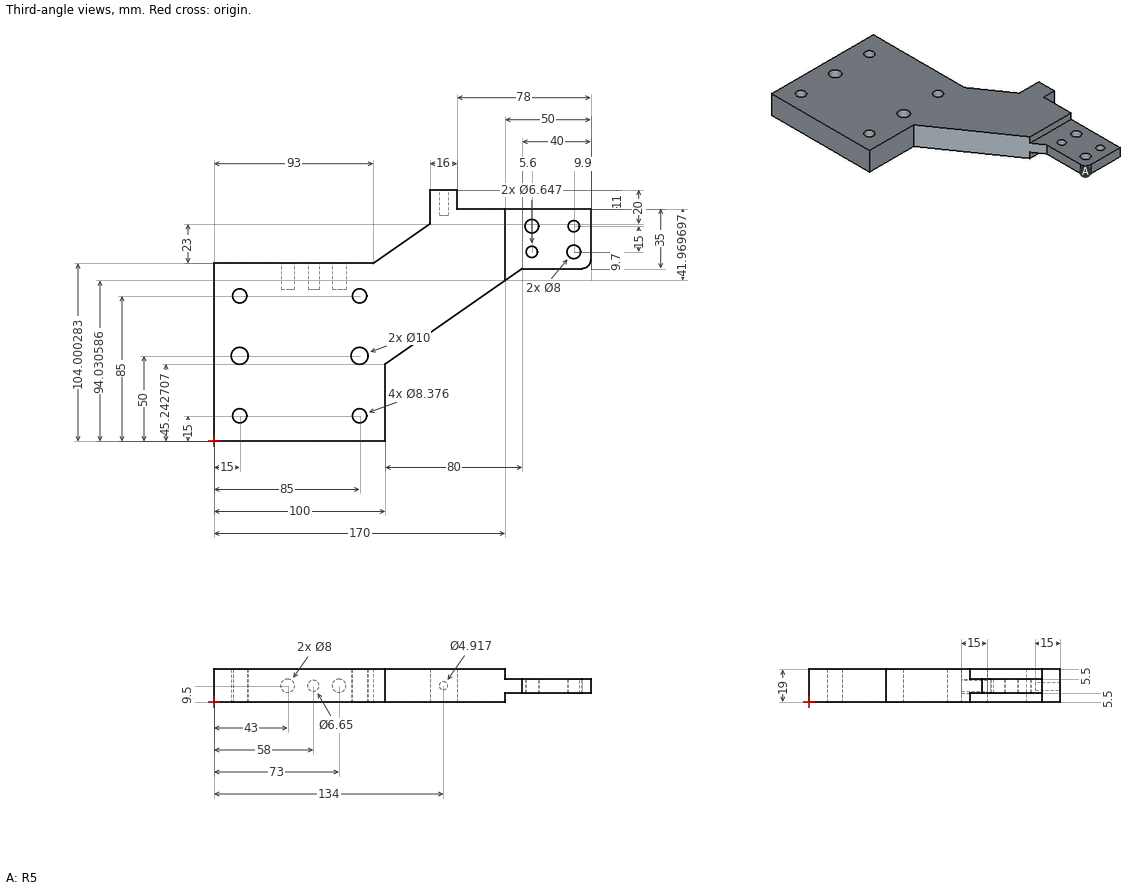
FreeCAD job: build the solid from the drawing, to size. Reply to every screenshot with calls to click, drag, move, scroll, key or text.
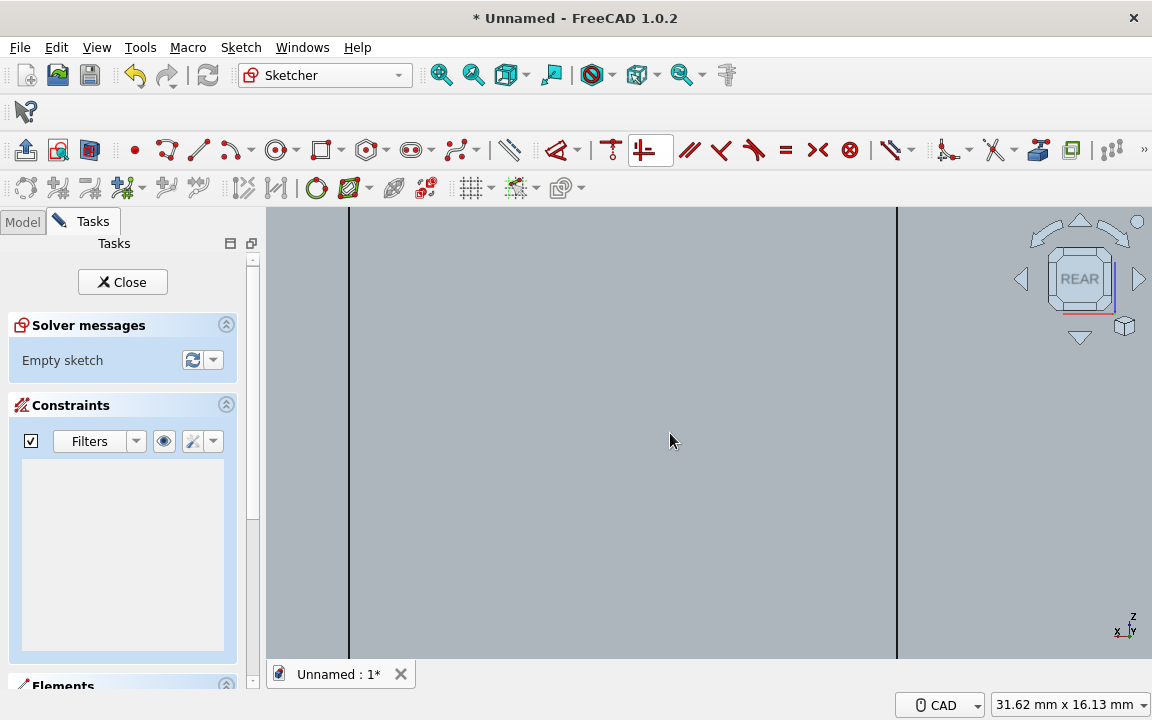
scroll(602, 412, up, 3)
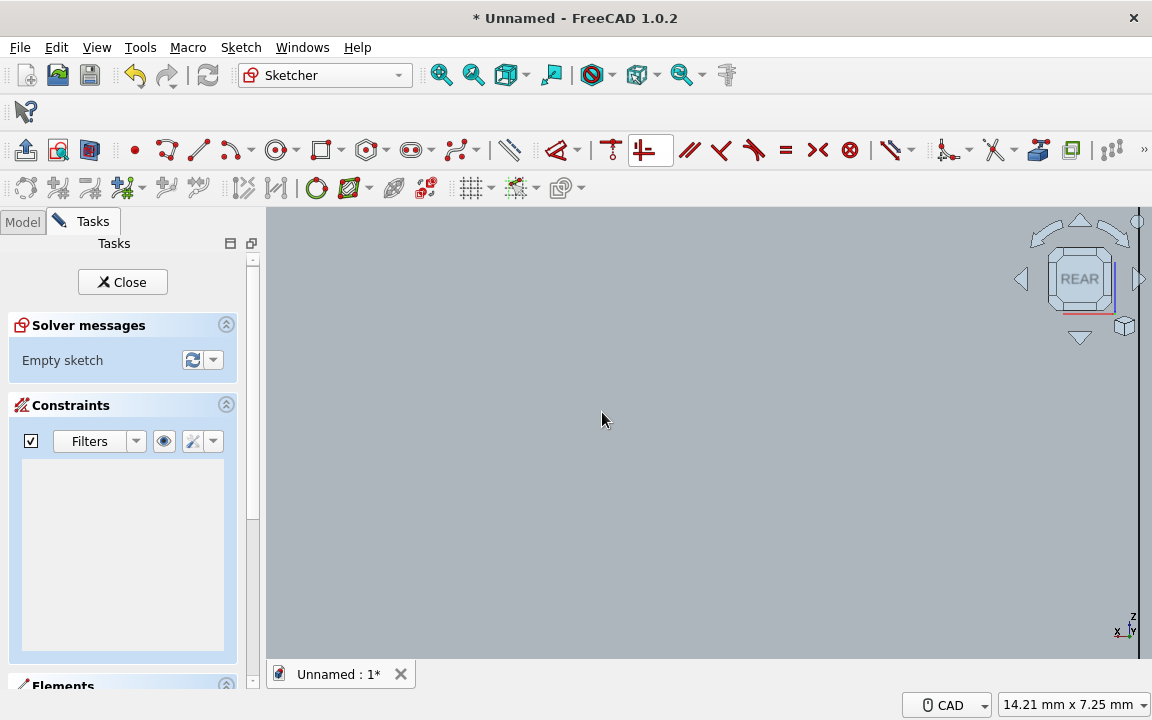
click(276, 150)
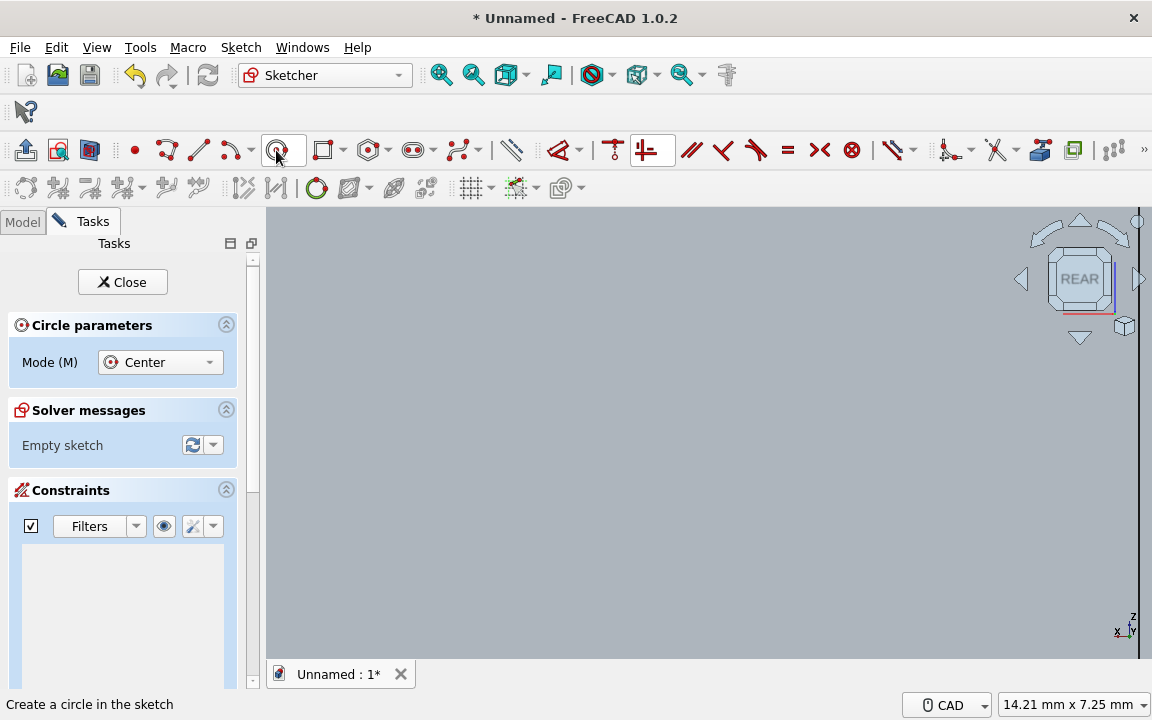
click(640, 432)
click(749, 324)
key(Escape)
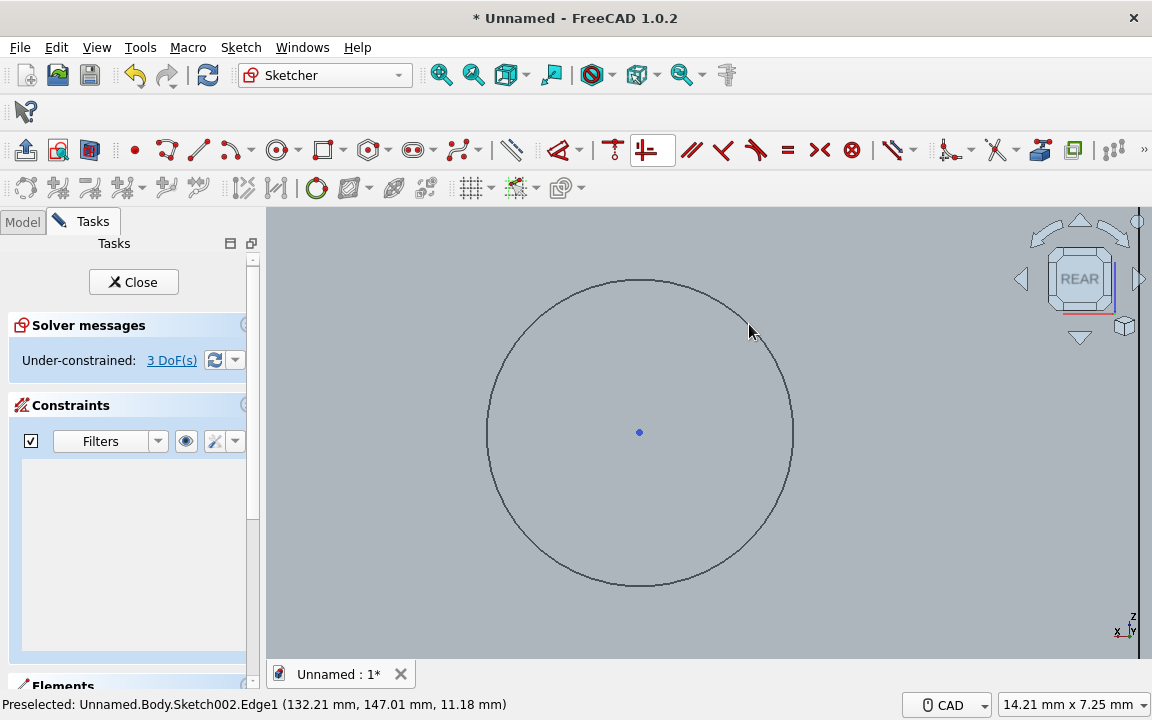
click(558, 150)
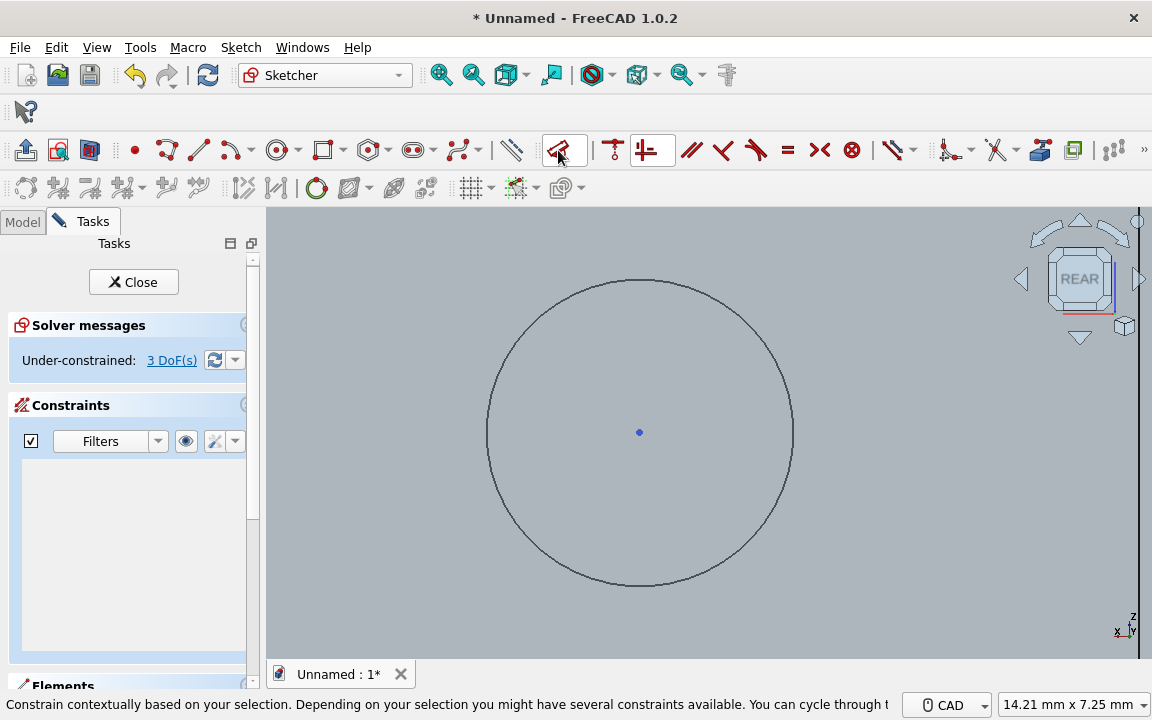
click(748, 324)
click(771, 301)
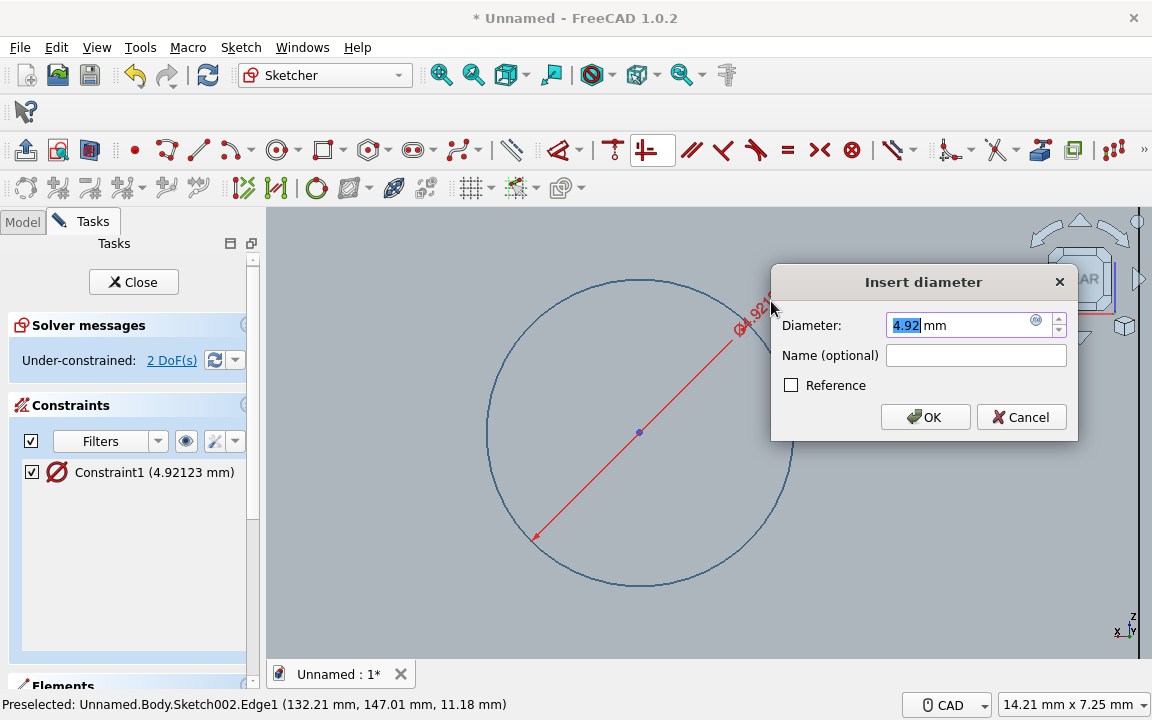
text(4.917)
key(Return)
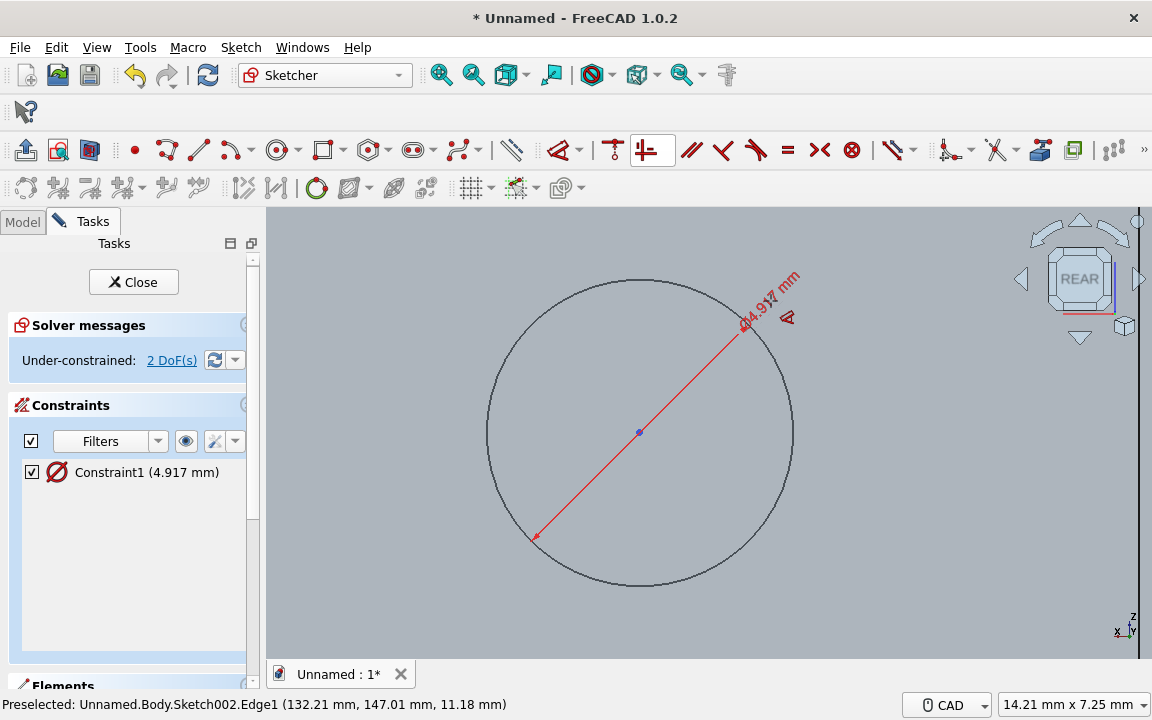
click(640, 433)
click(814, 399)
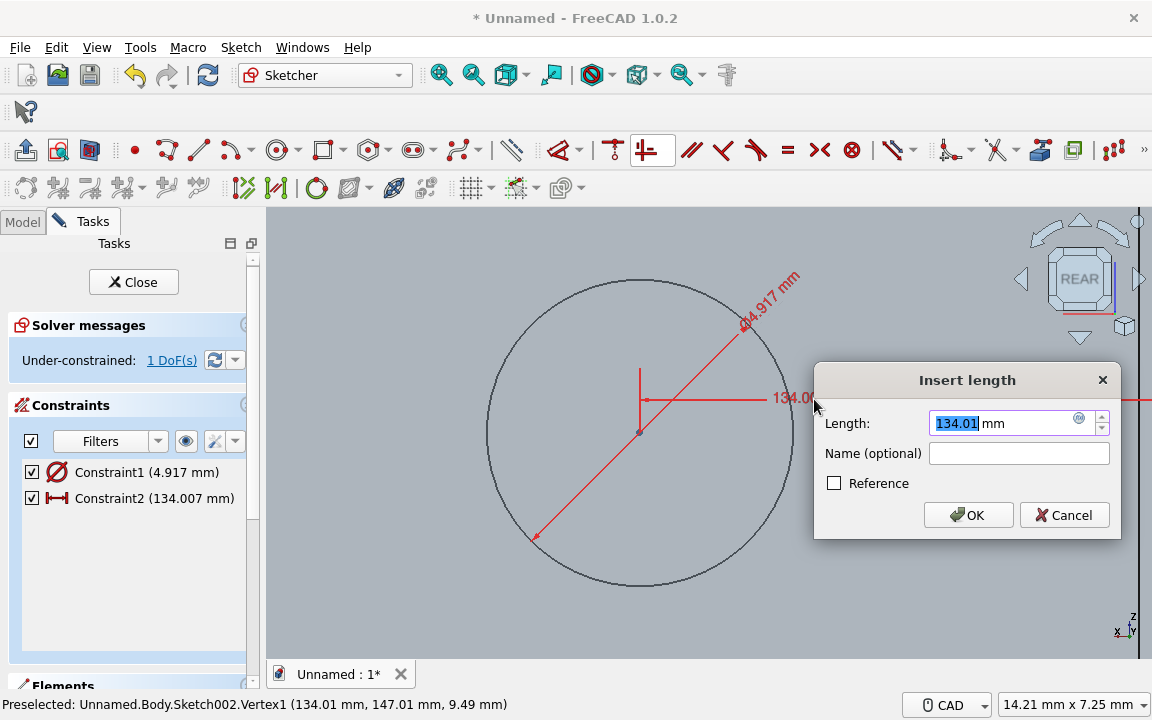
text(134)
key(Return)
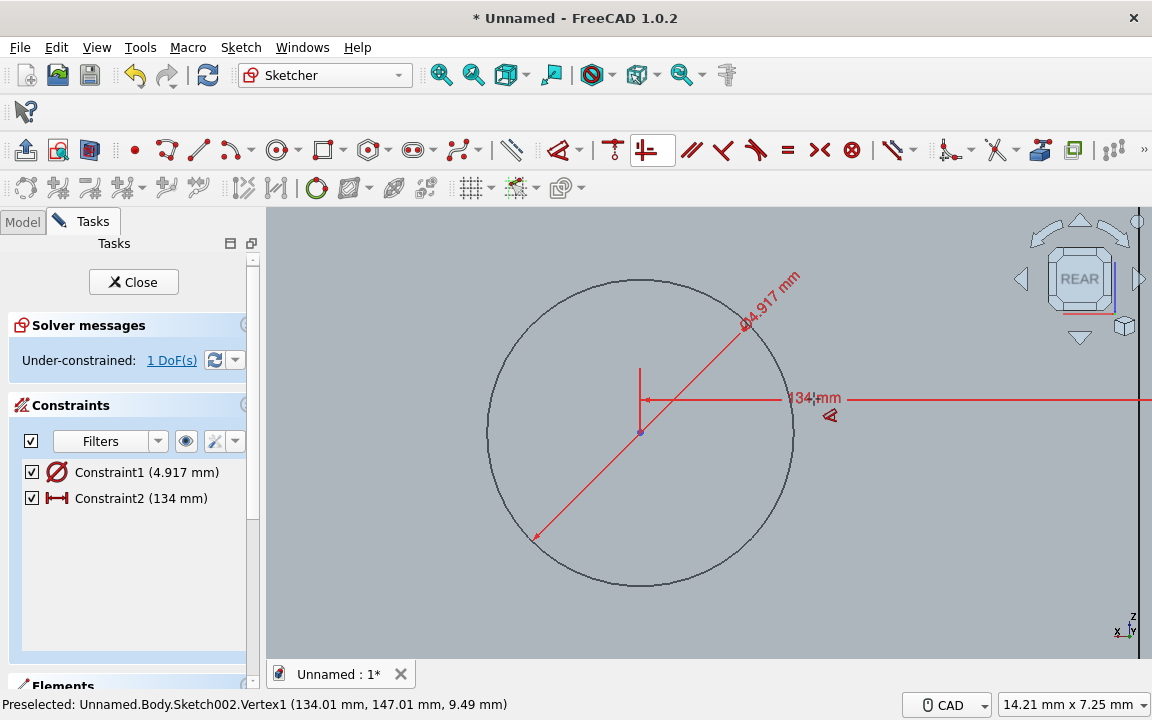
click(640, 433)
click(606, 532)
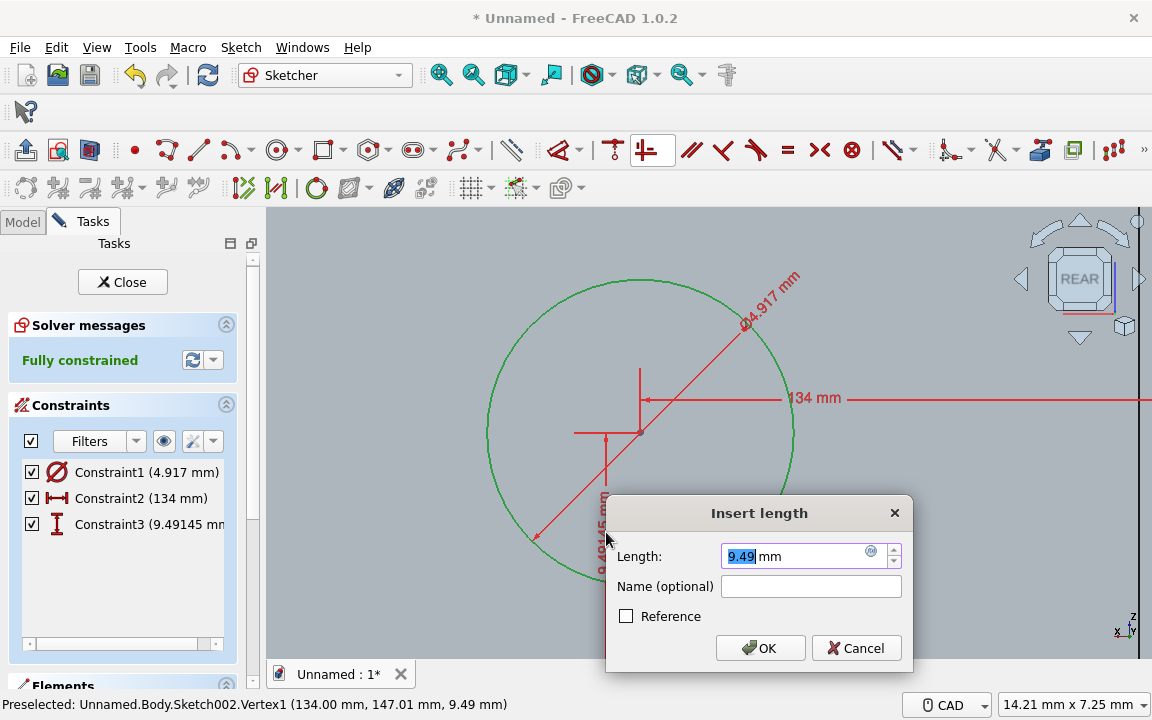
text(9.5)
key(Return)
key(Escape)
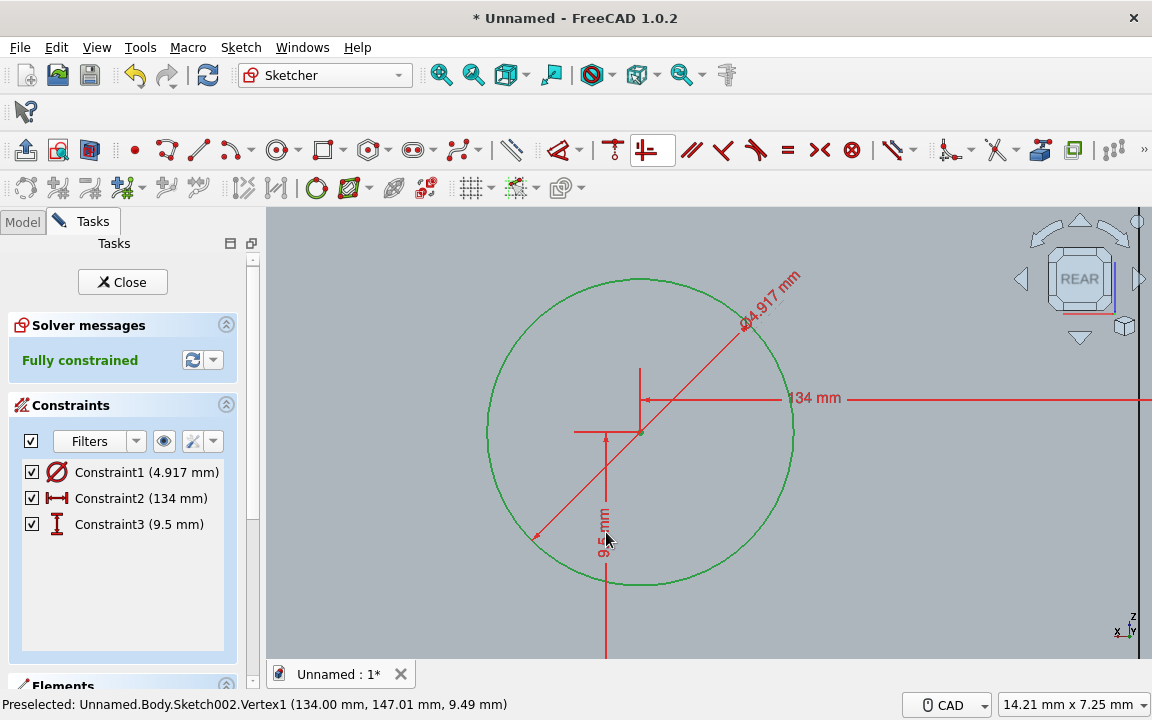
click(123, 282)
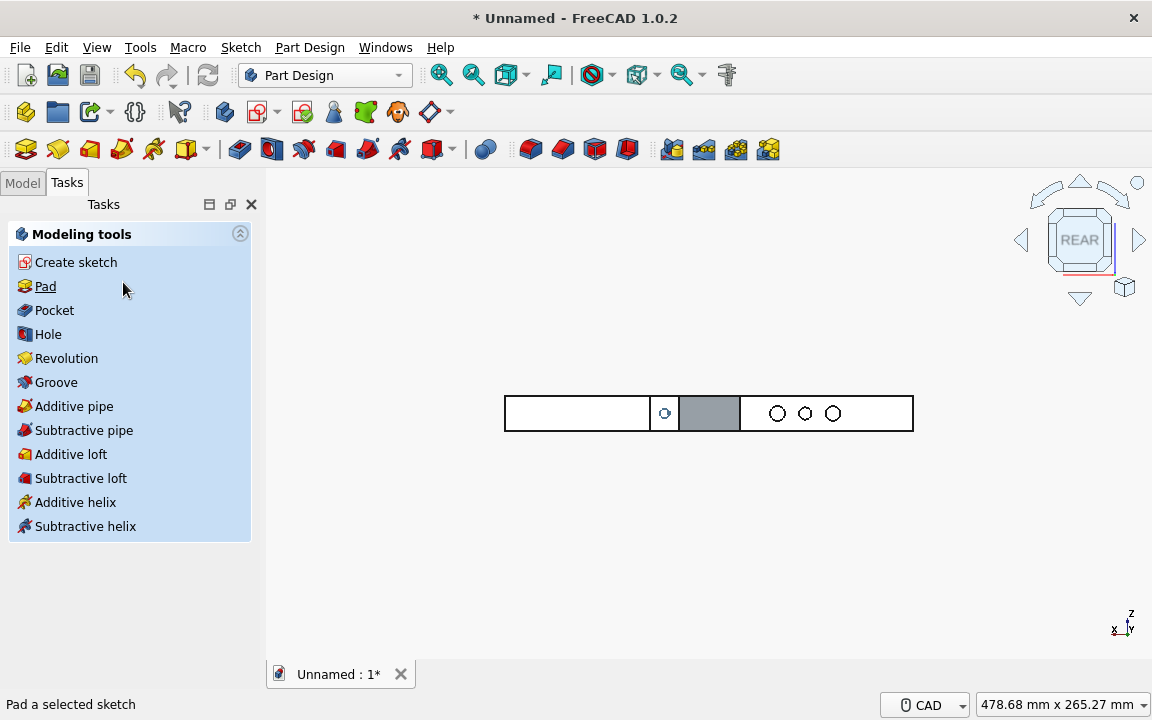
click(240, 150)